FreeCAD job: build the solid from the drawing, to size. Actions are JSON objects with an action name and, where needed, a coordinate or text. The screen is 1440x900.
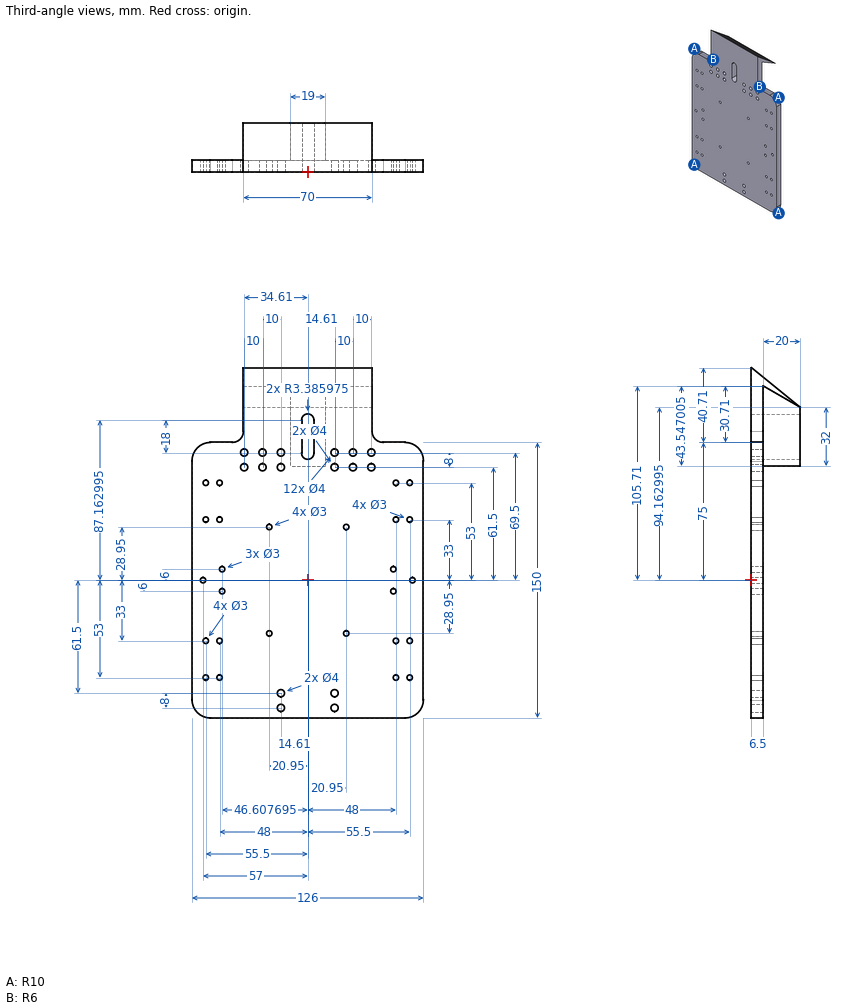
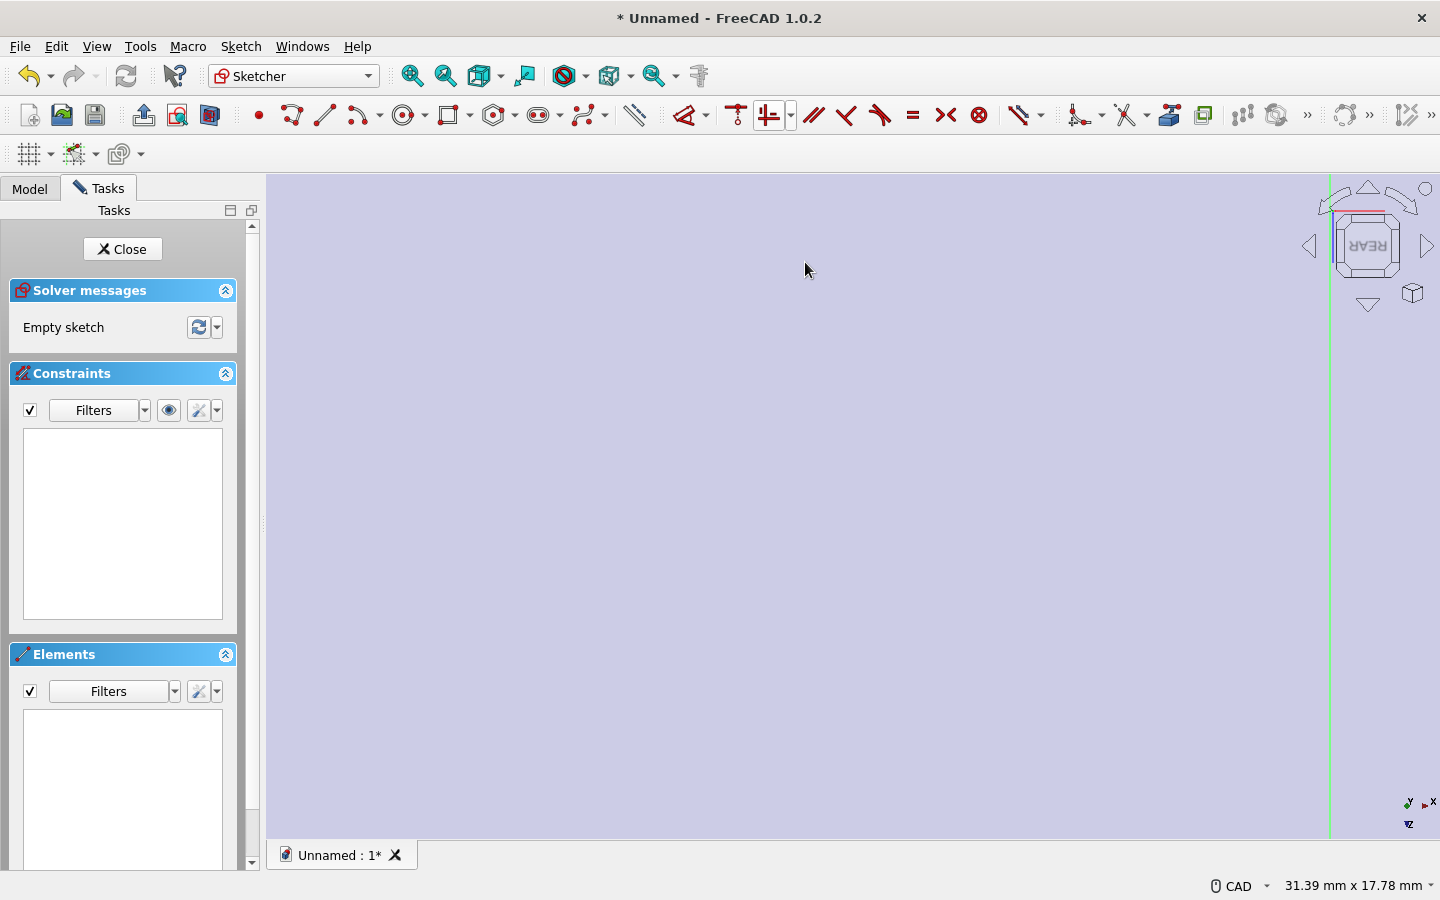
{"action": "left_click", "coordinate": [402, 116]}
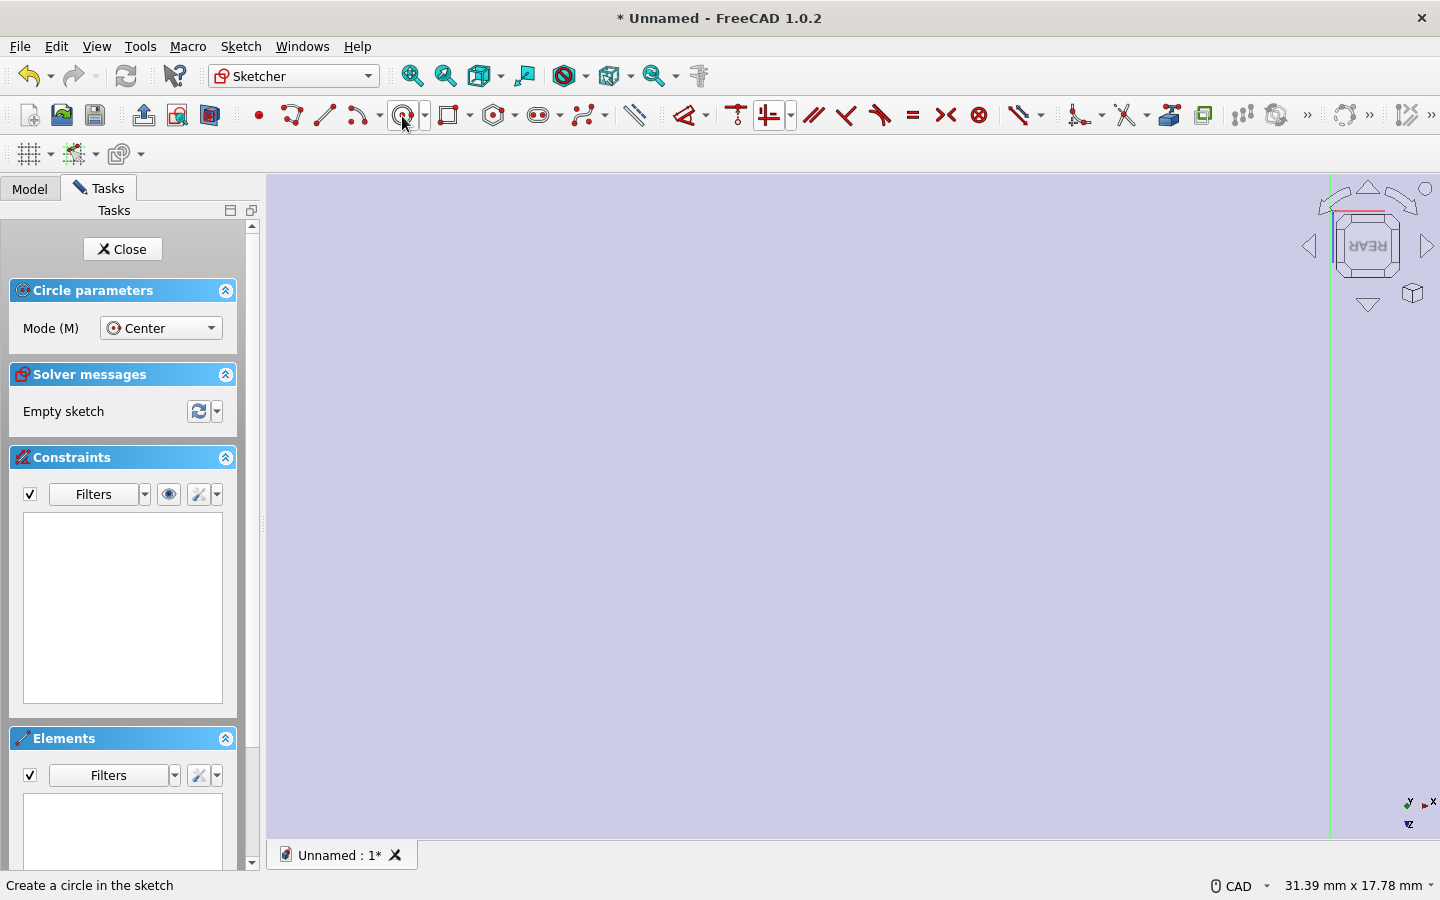
{"action": "left_click", "coordinate": [783, 656]}
{"action": "mouse_move", "coordinate": [836, 603]}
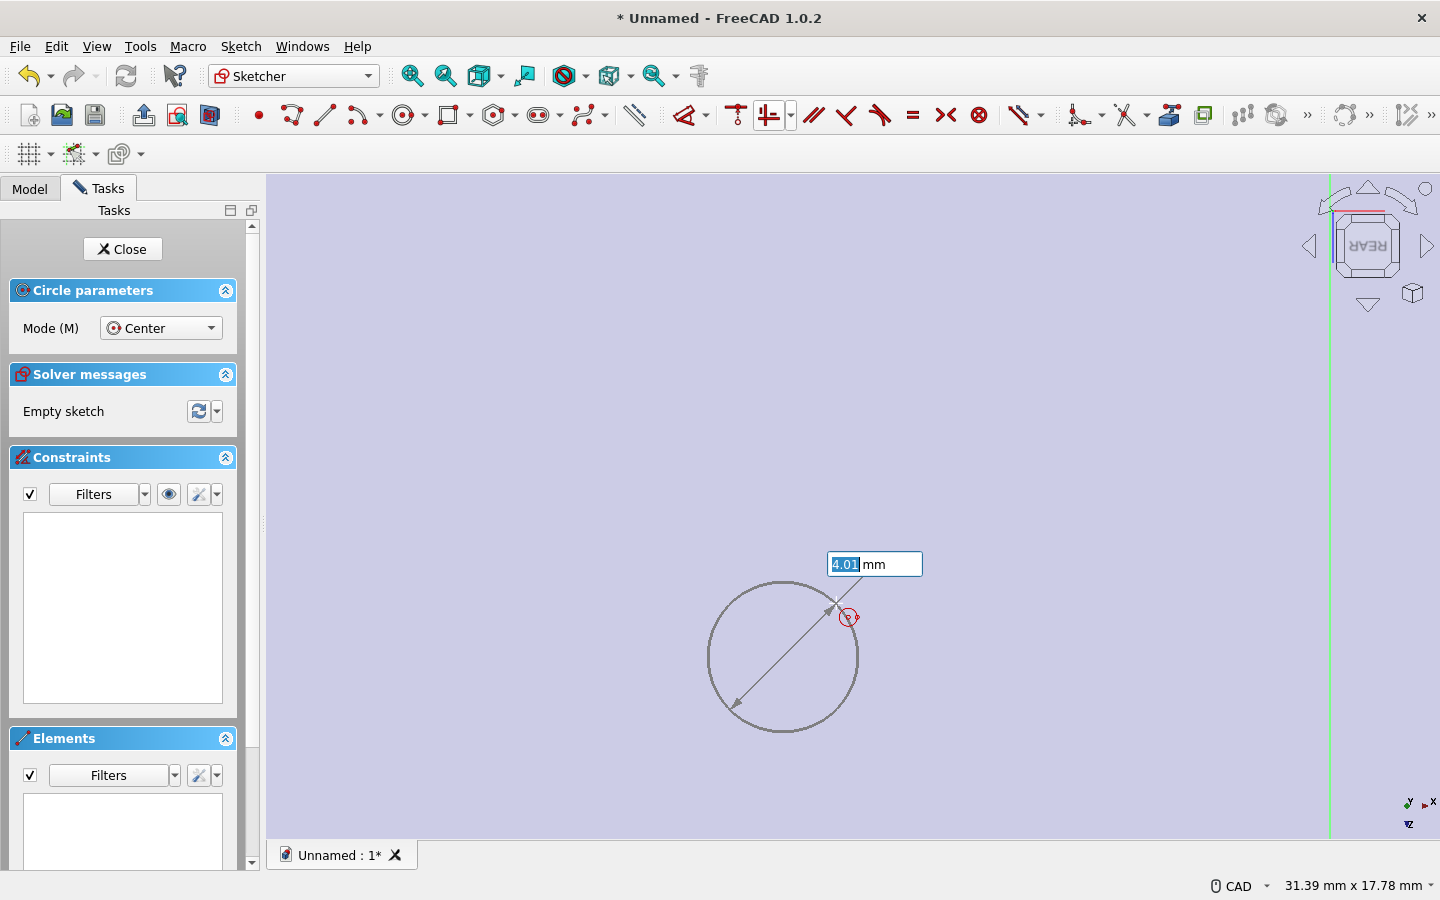
{"action": "type", "text": "4"}
{"action": "key", "text": "Return"}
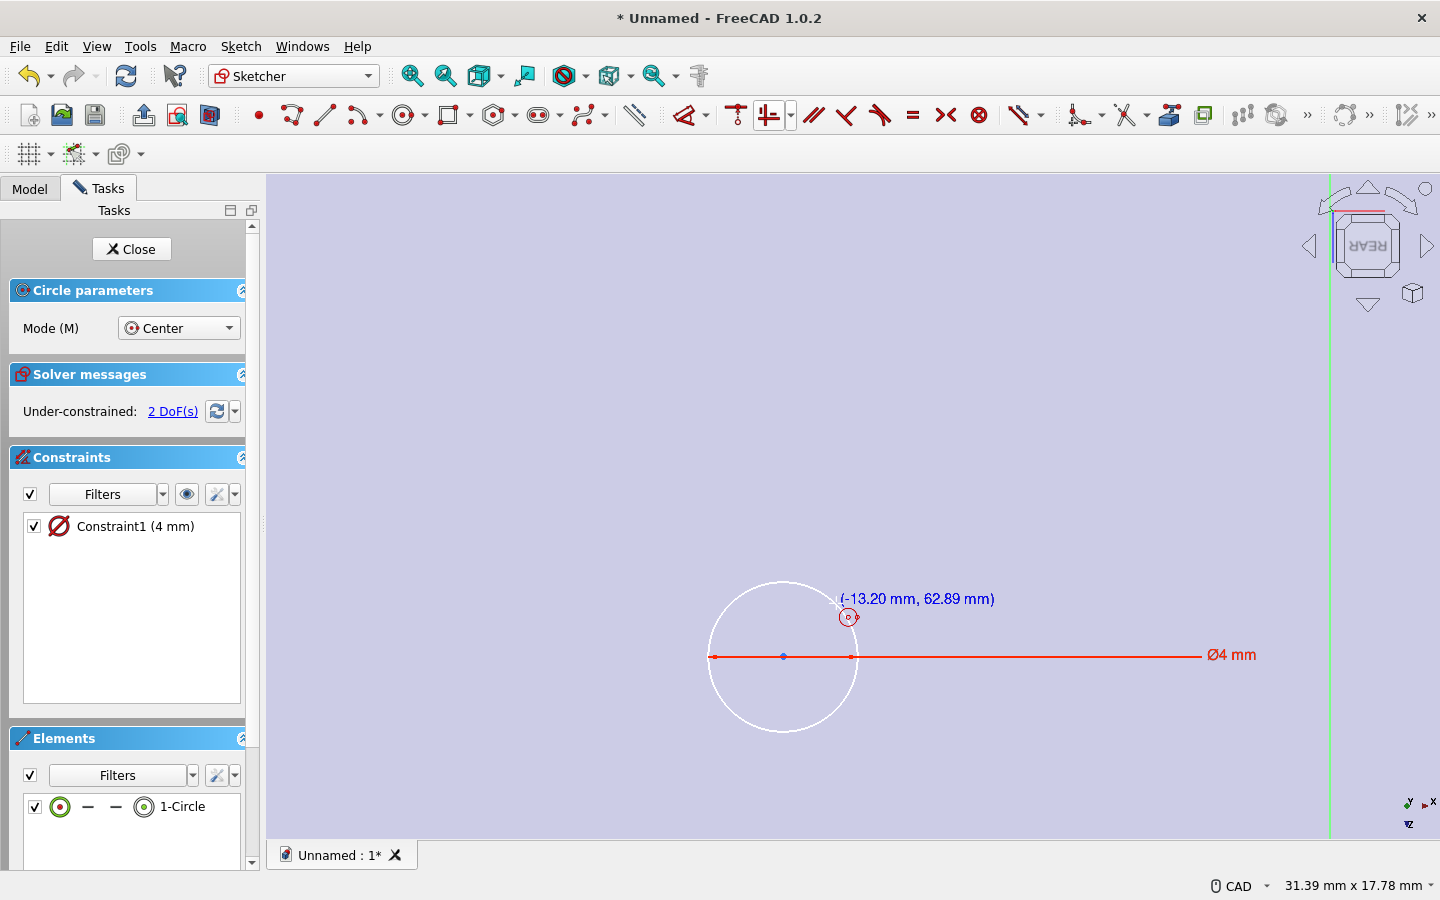
{"action": "left_click", "coordinate": [783, 357]}
{"action": "mouse_move", "coordinate": [836, 304]}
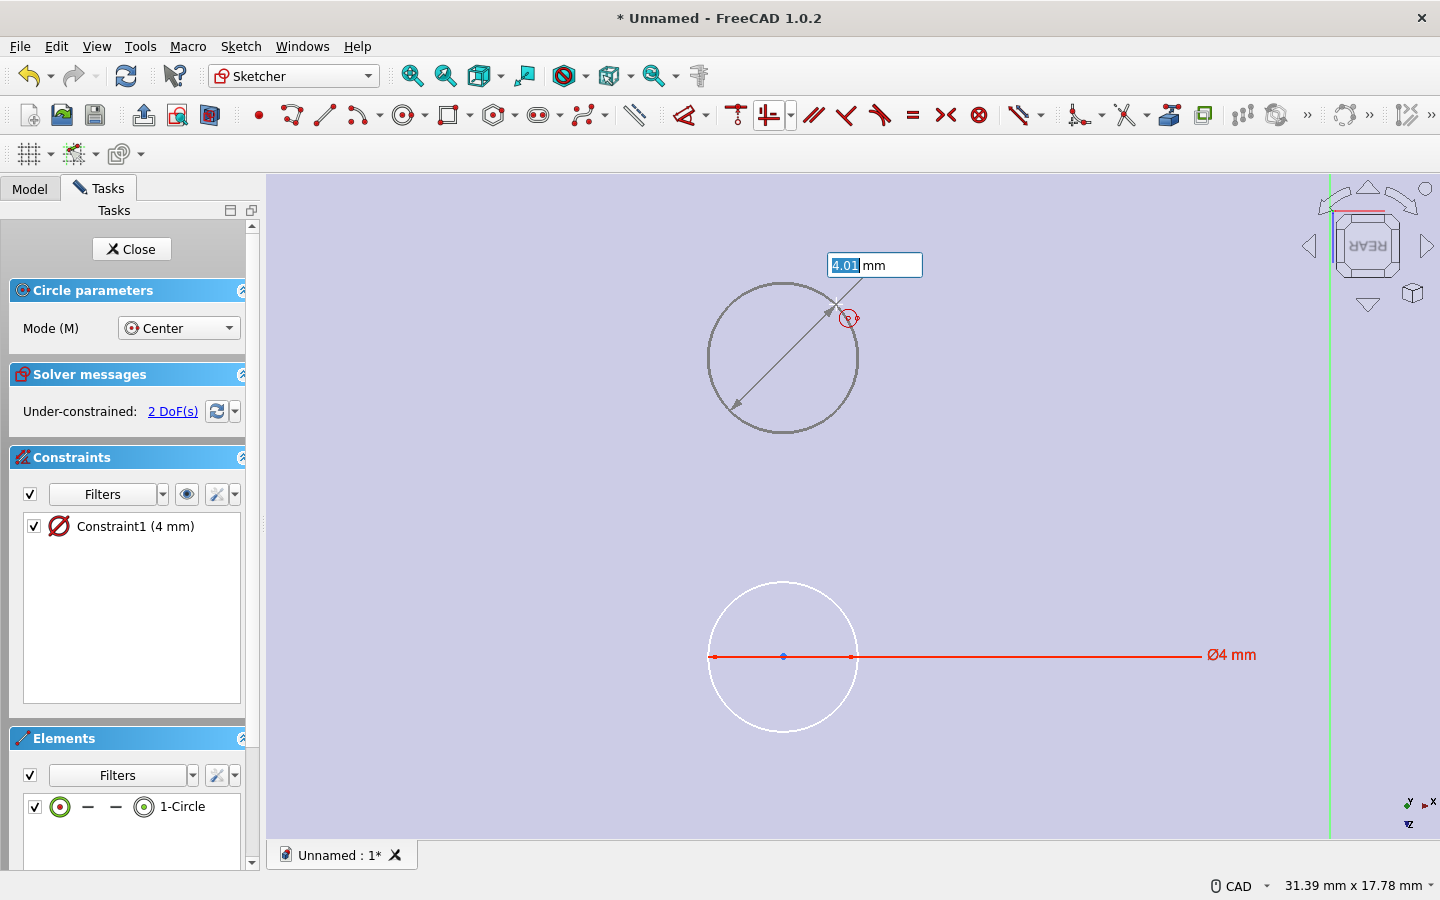
{"action": "type", "text": "4"}
{"action": "key", "text": "Return"}
{"action": "key", "text": "Escape"}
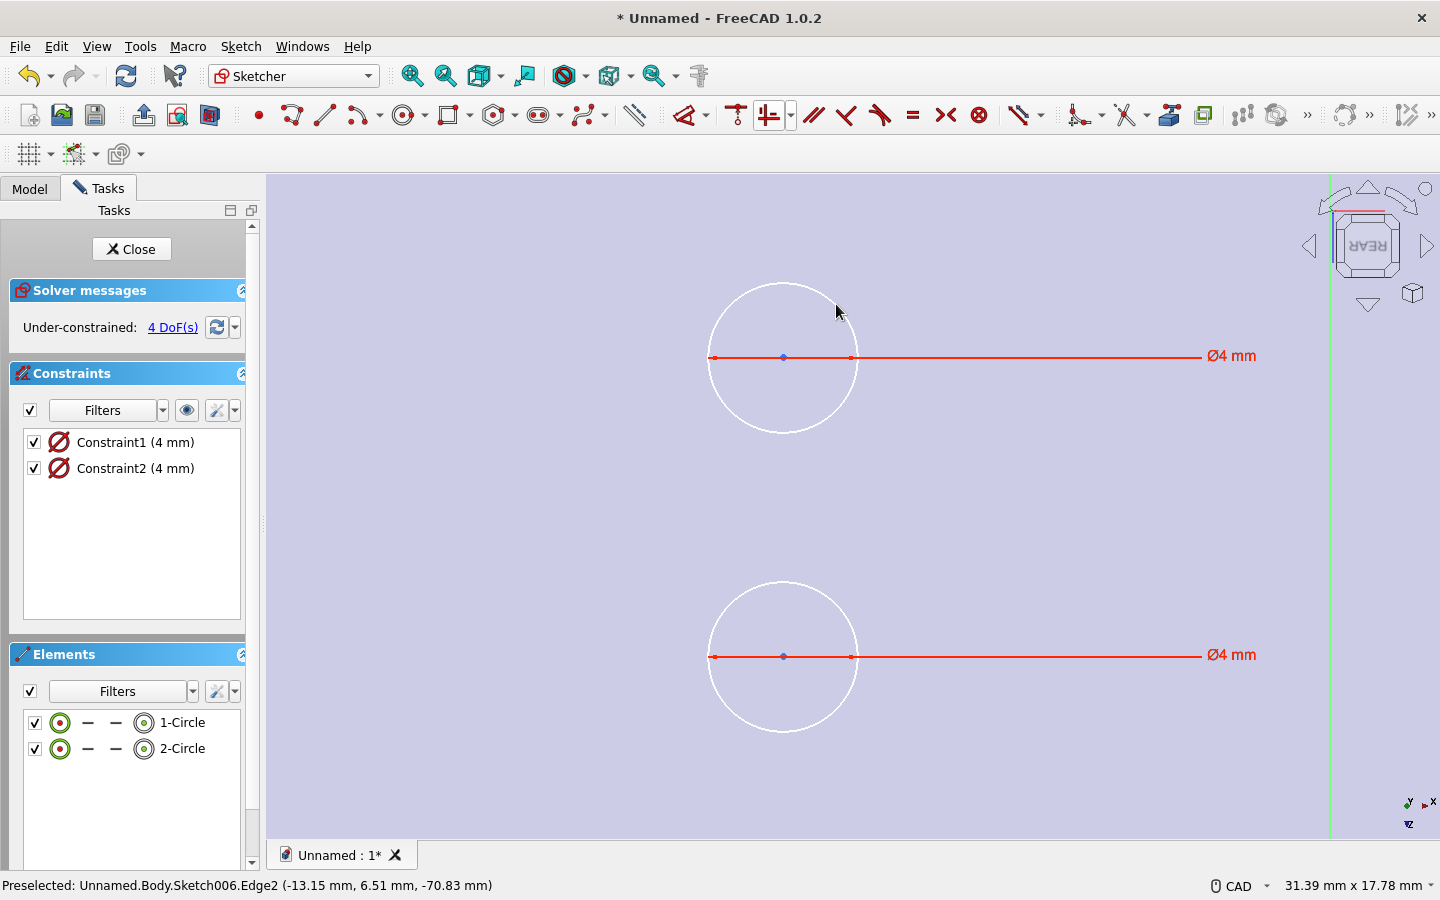
{"action": "left_click", "coordinate": [783, 657]}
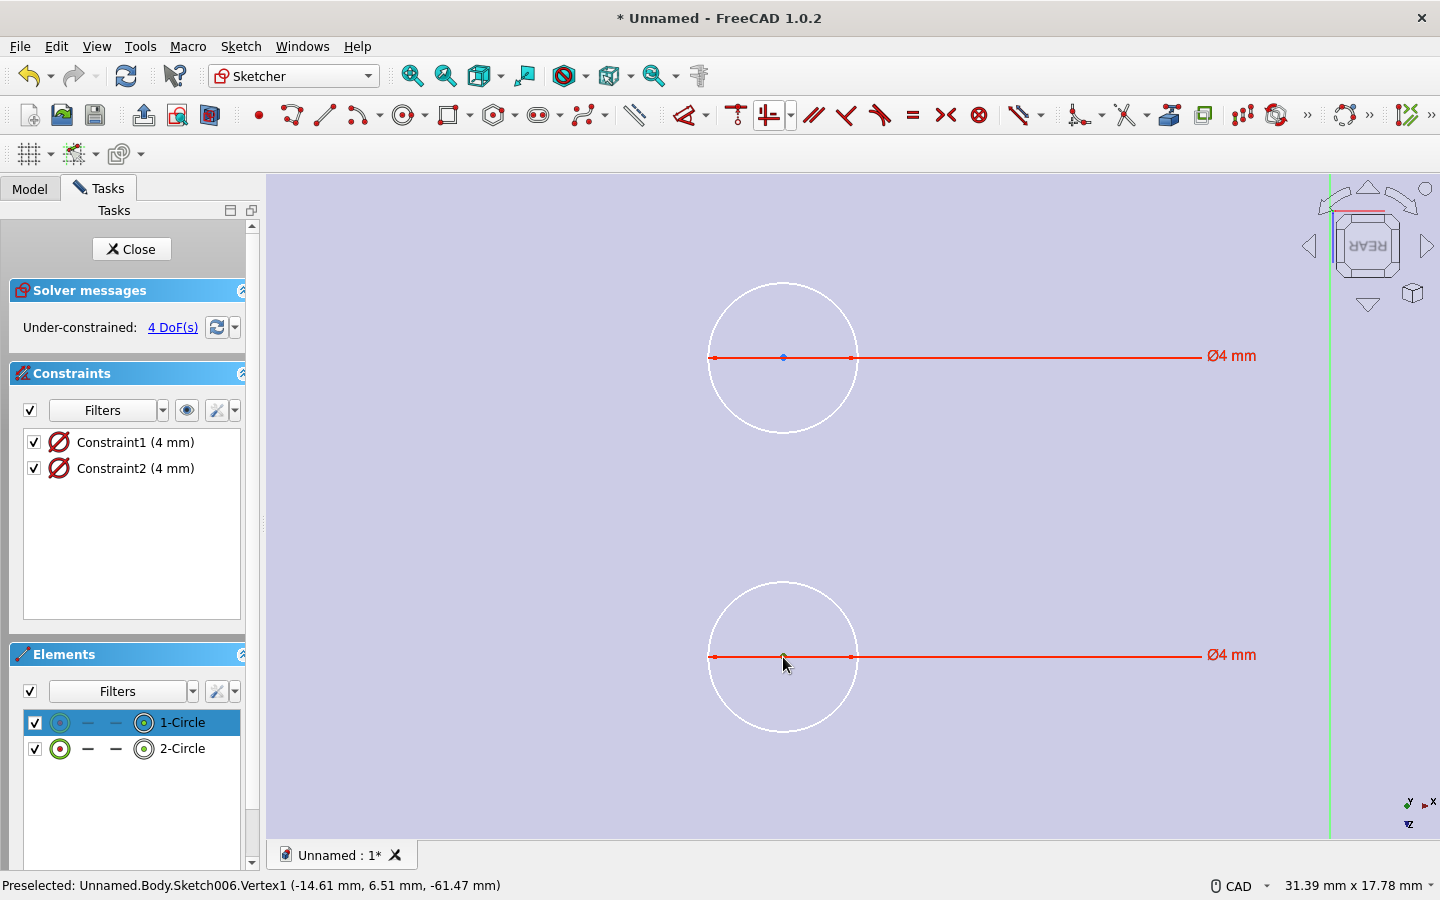
{"action": "left_click", "coordinate": [783, 358]}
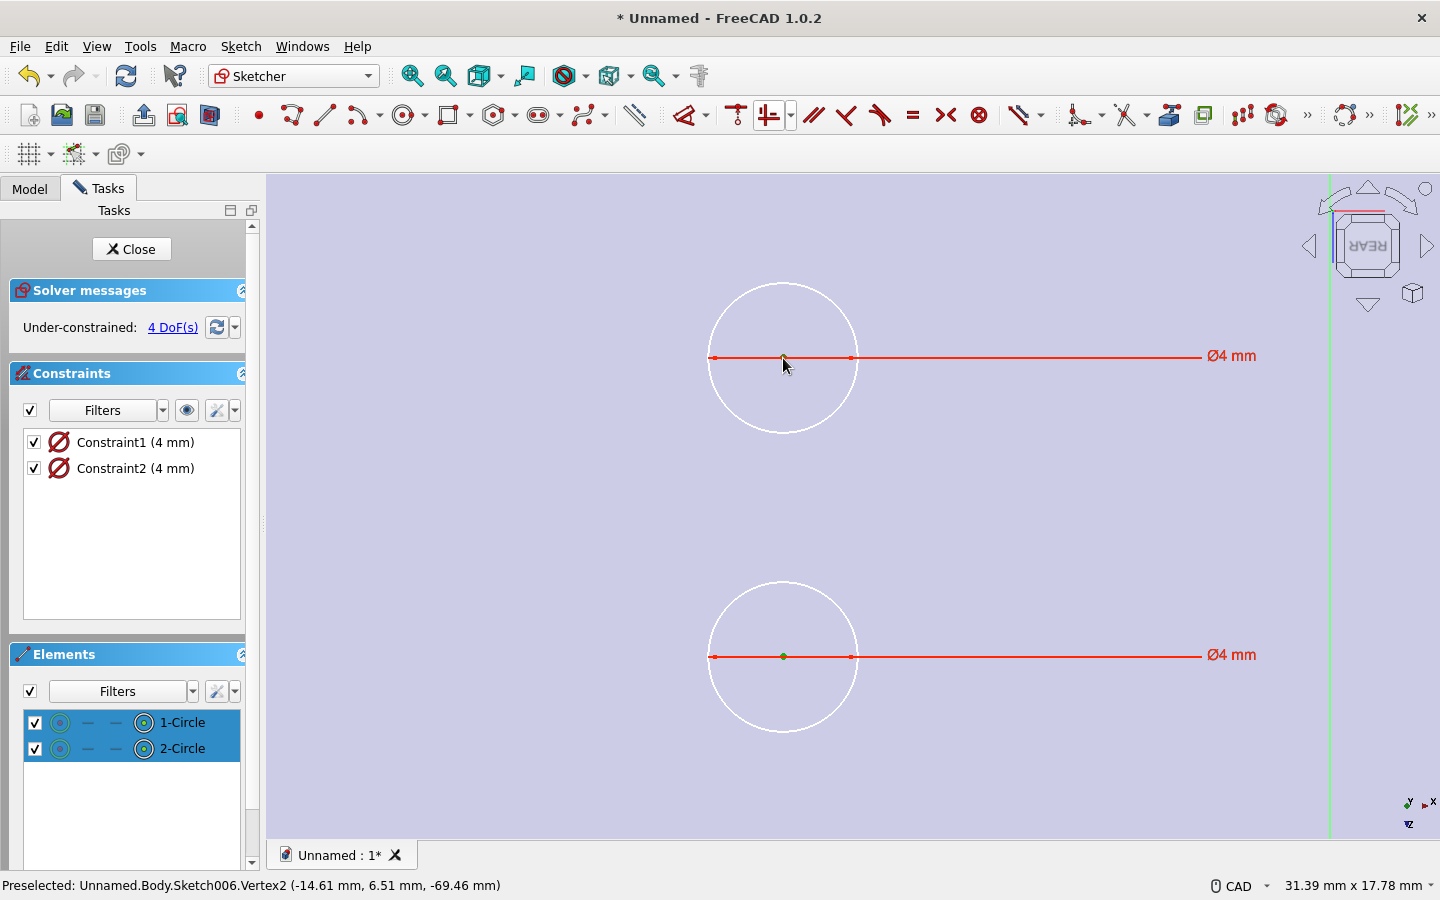
{"action": "key", "text": "v"}